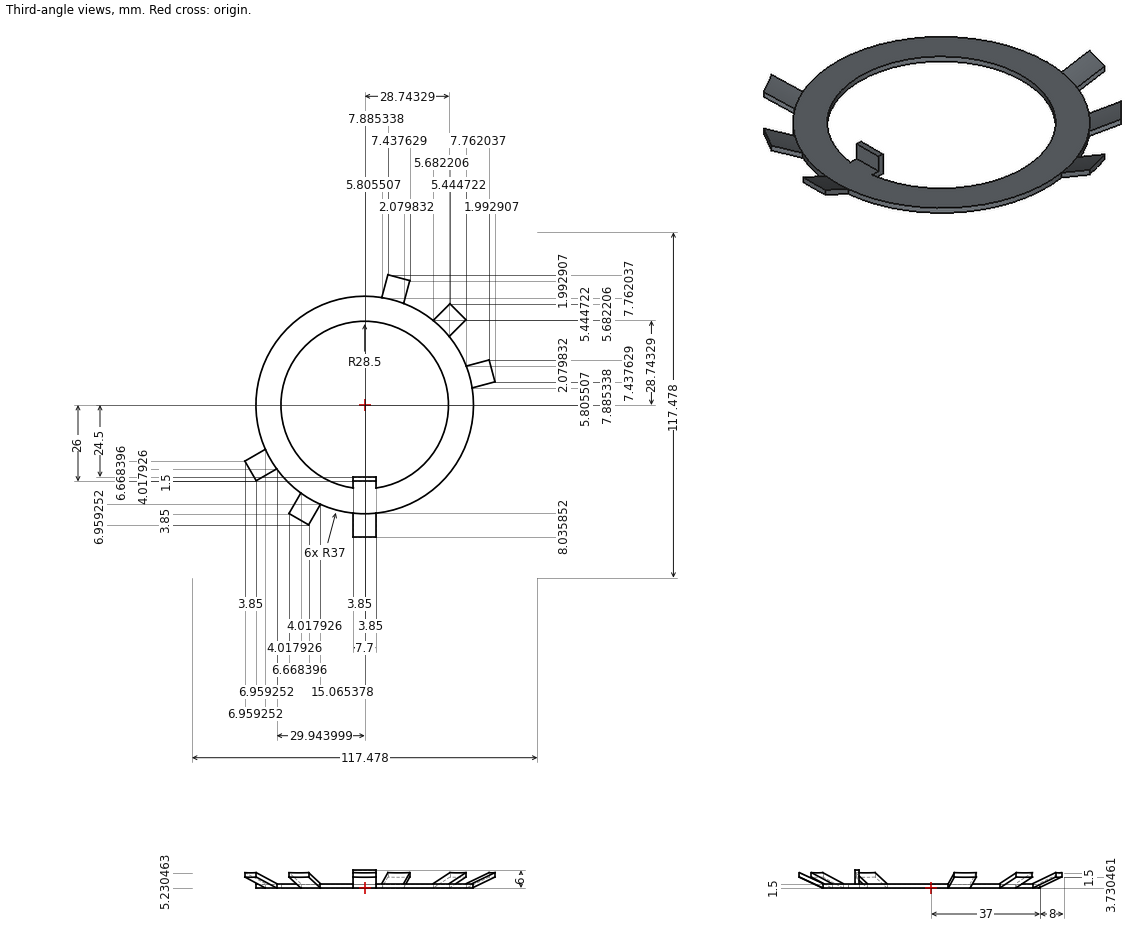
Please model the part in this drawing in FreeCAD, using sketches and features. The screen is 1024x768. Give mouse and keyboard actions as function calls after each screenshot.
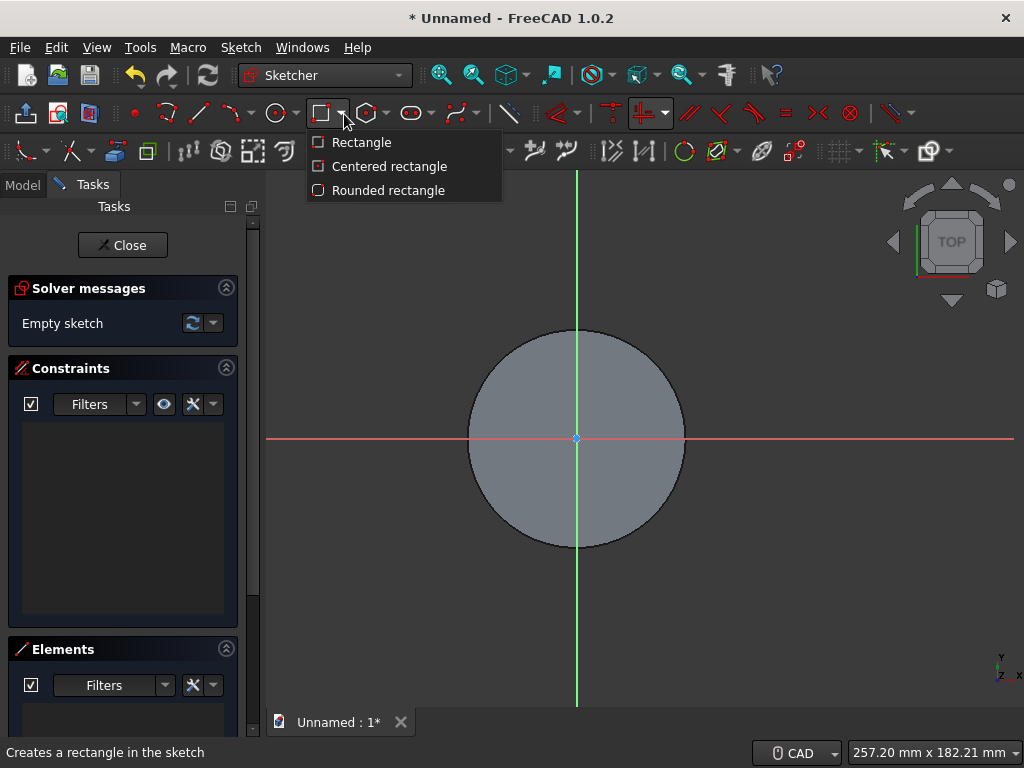
click(404, 166)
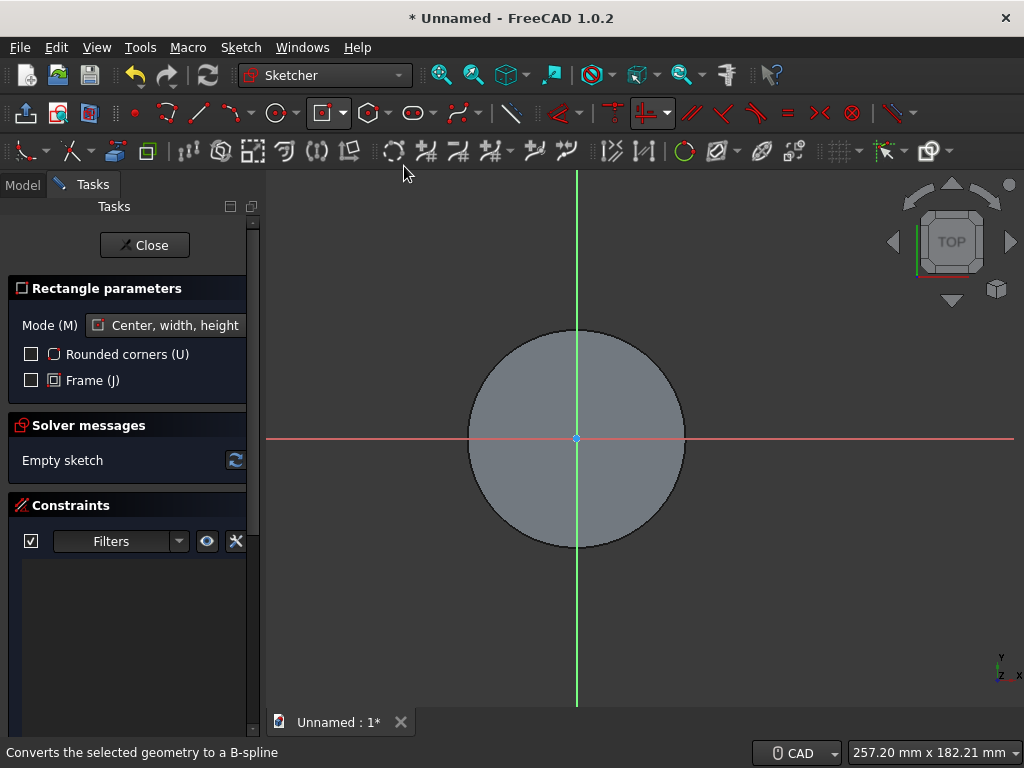
click(577, 439)
click(750, 266)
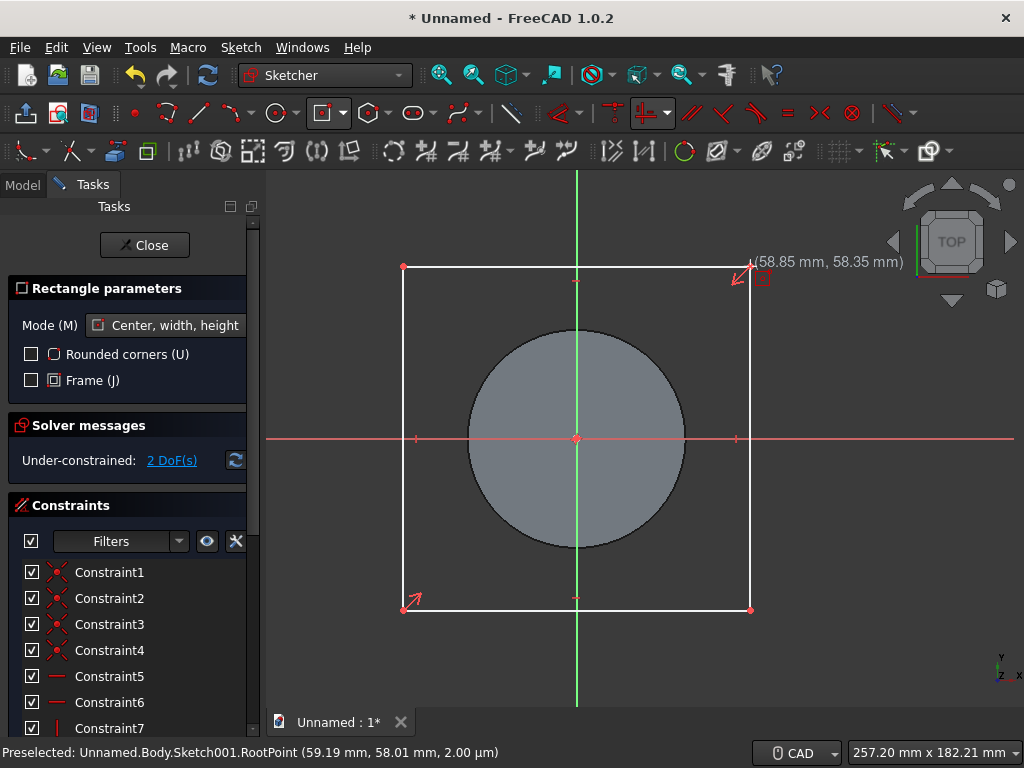
click(168, 114)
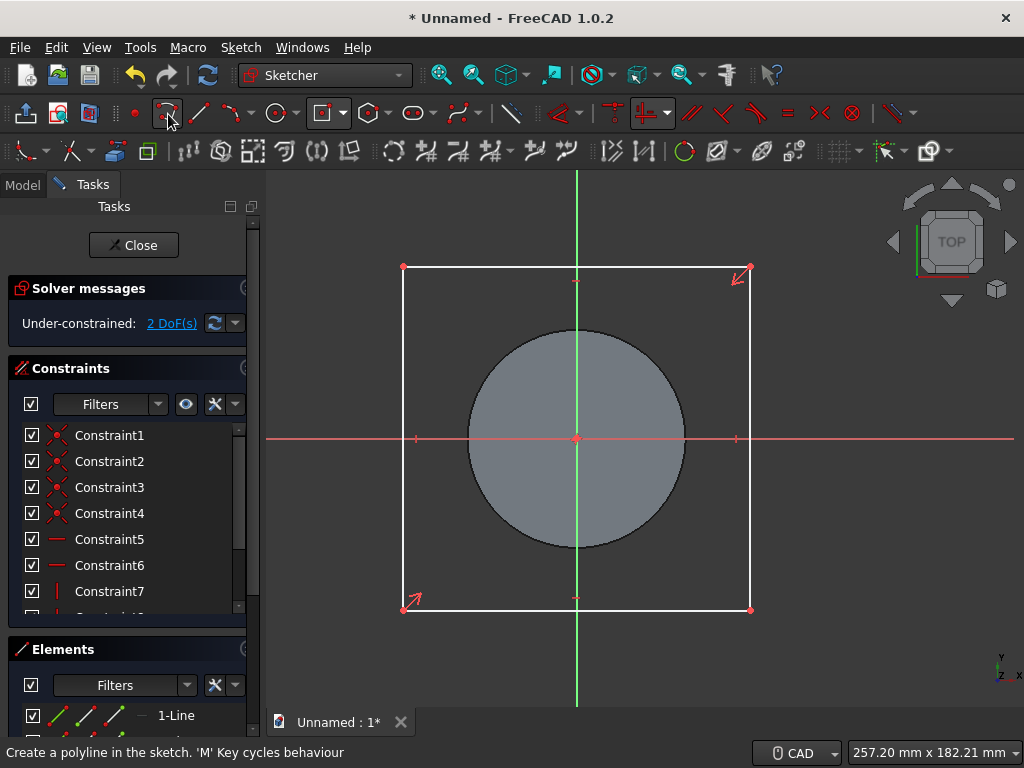
scroll(565, 522, up, 2)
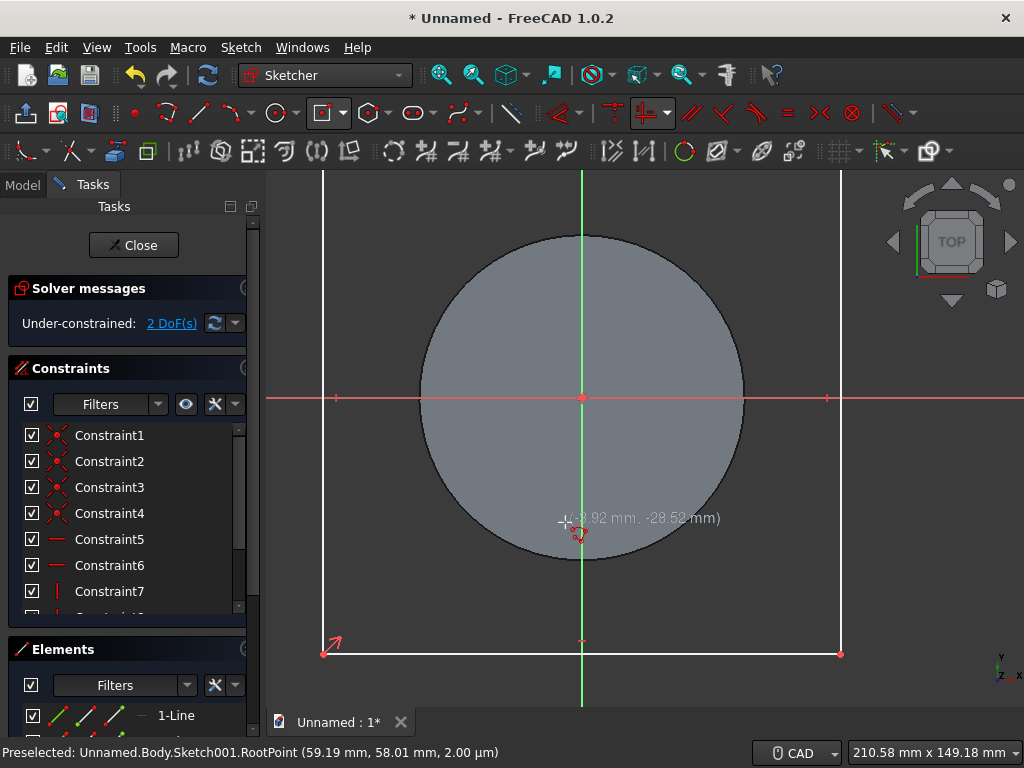
click(565, 522)
click(565, 506)
click(599, 506)
click(599, 522)
right_click(599, 522)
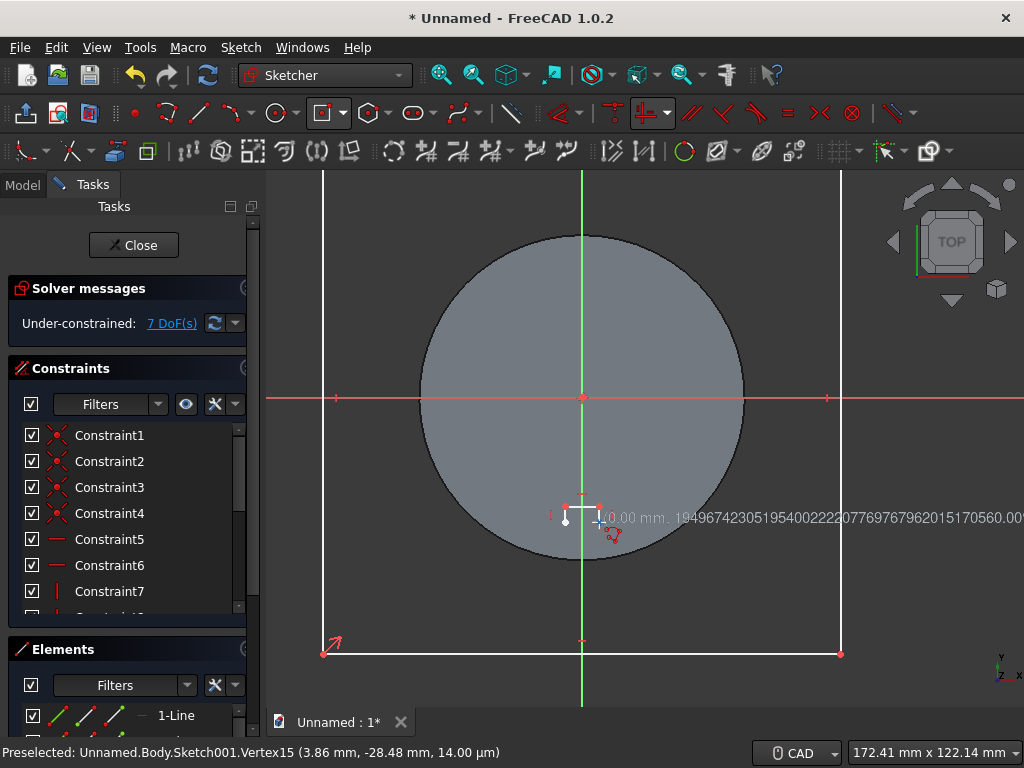
click(232, 114)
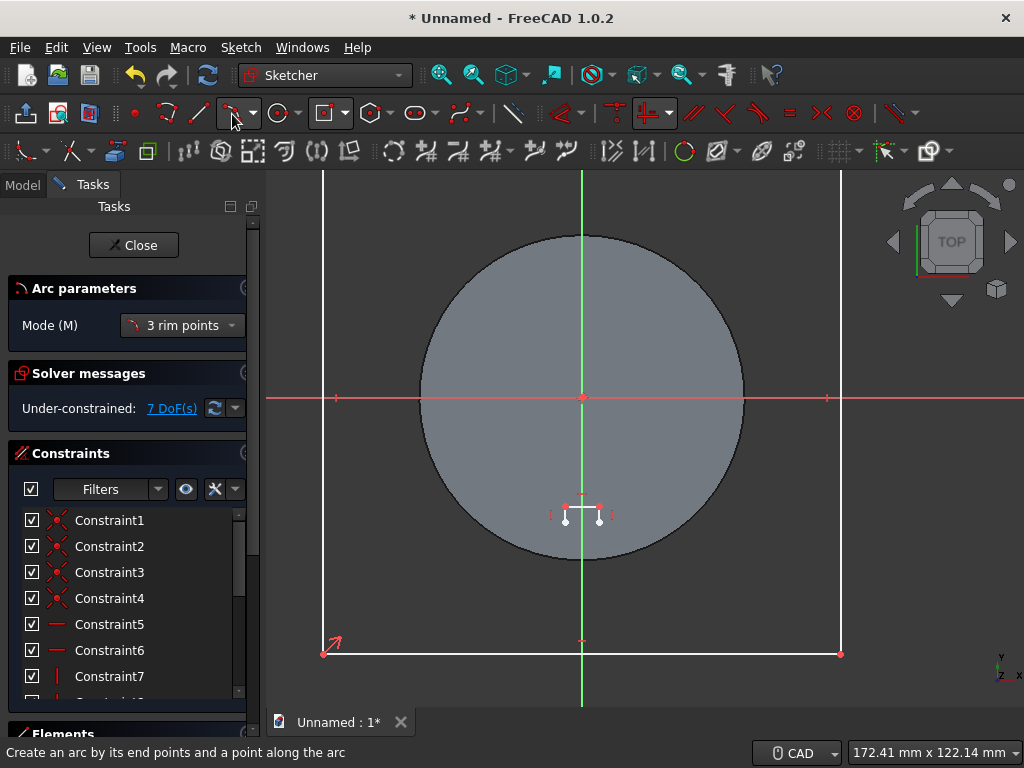
scroll(599, 522, up, 4)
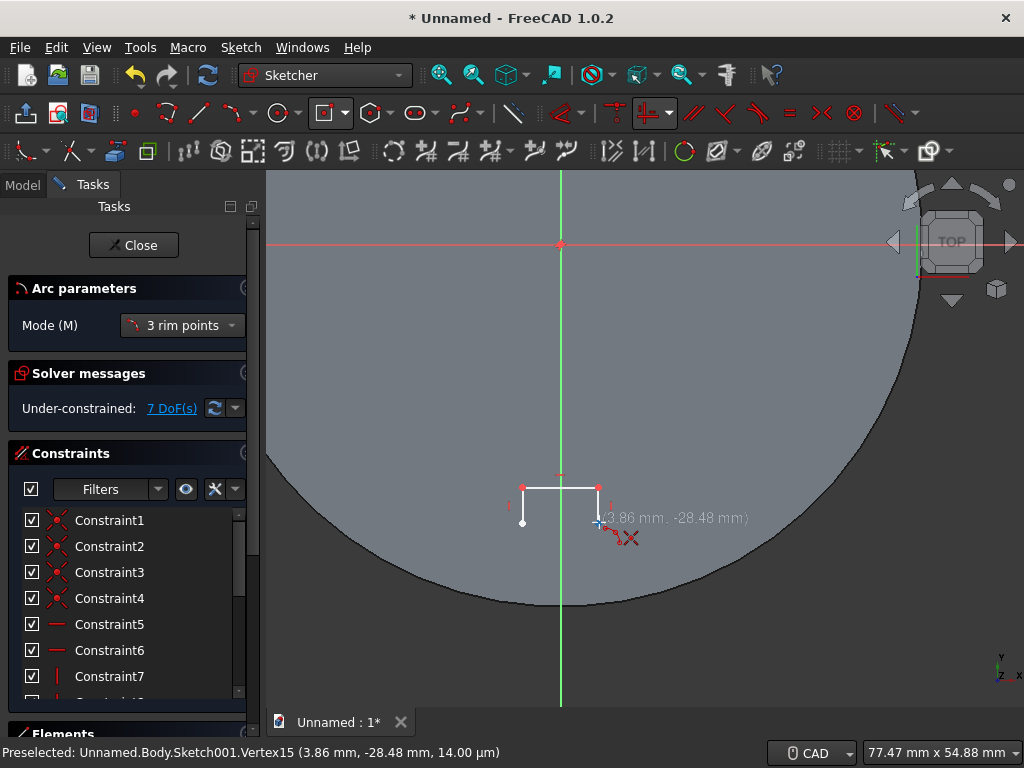
click(598, 523)
click(523, 523)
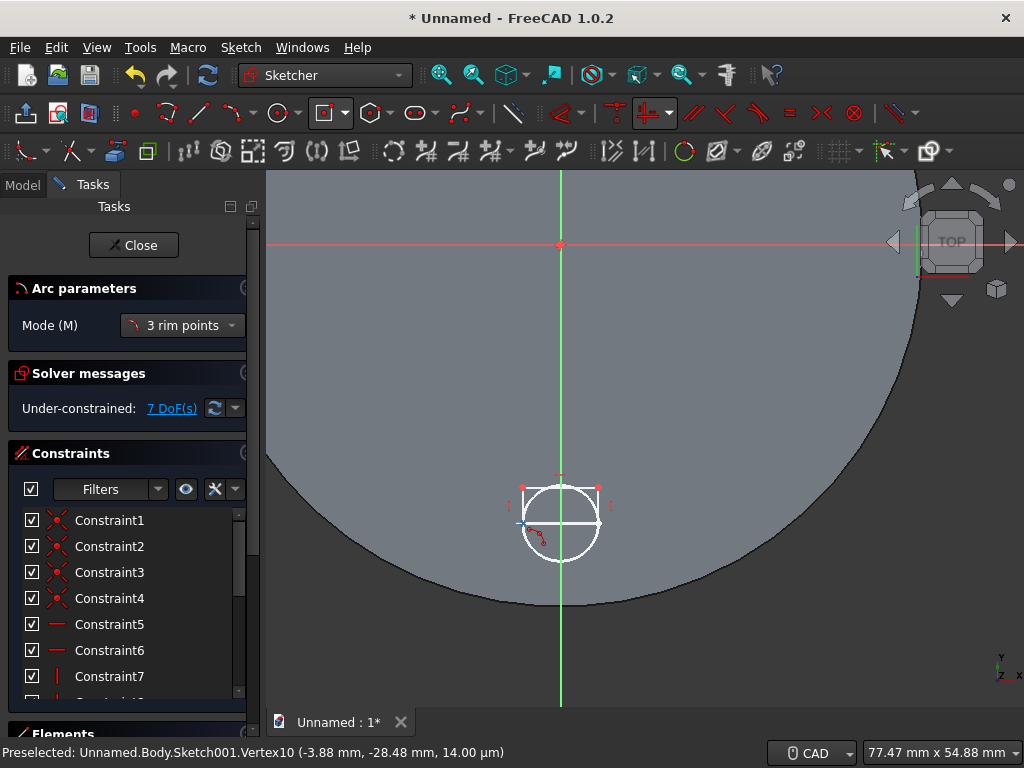
scroll(583, 522, down, 6)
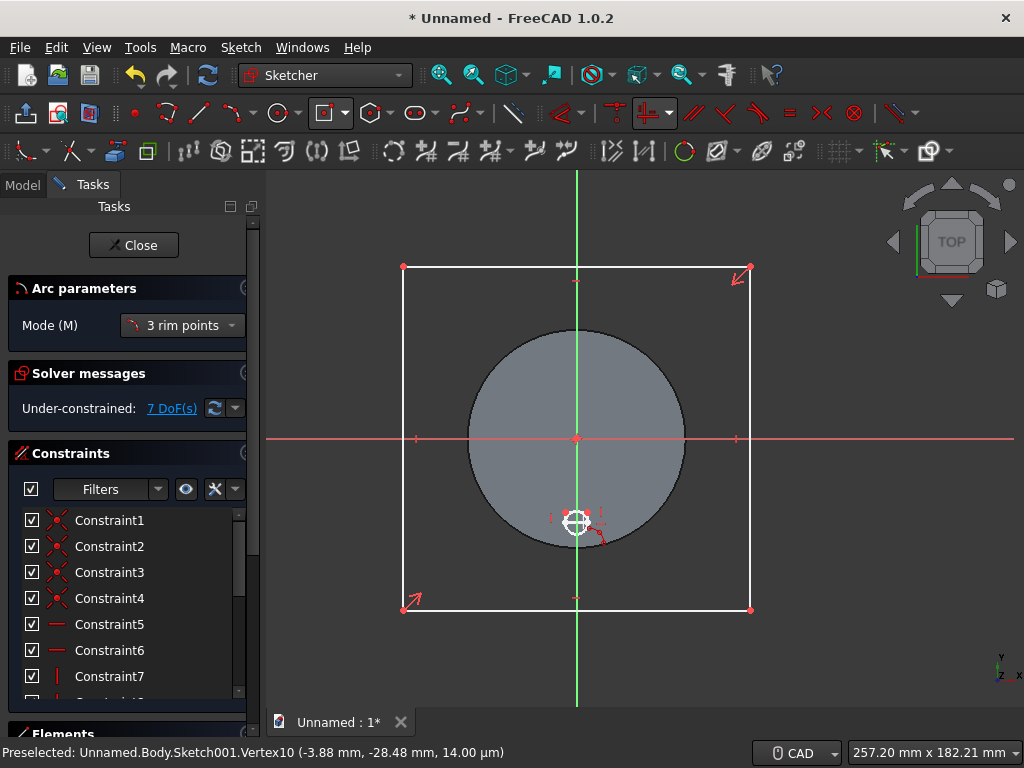
click(624, 370)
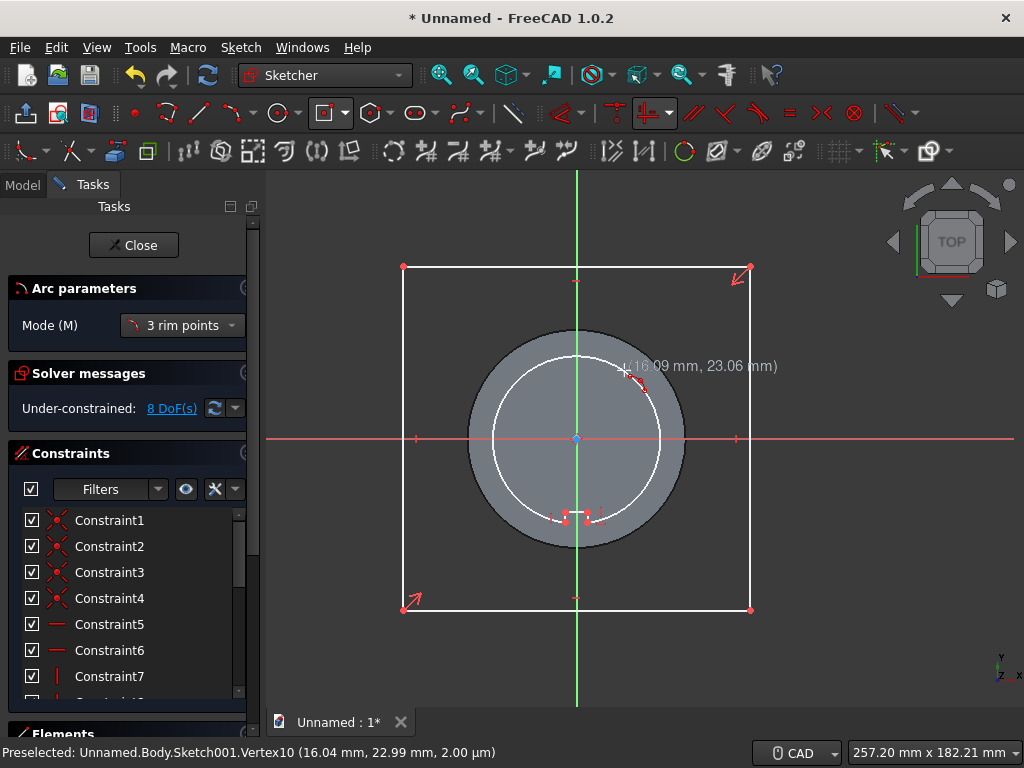
click(168, 114)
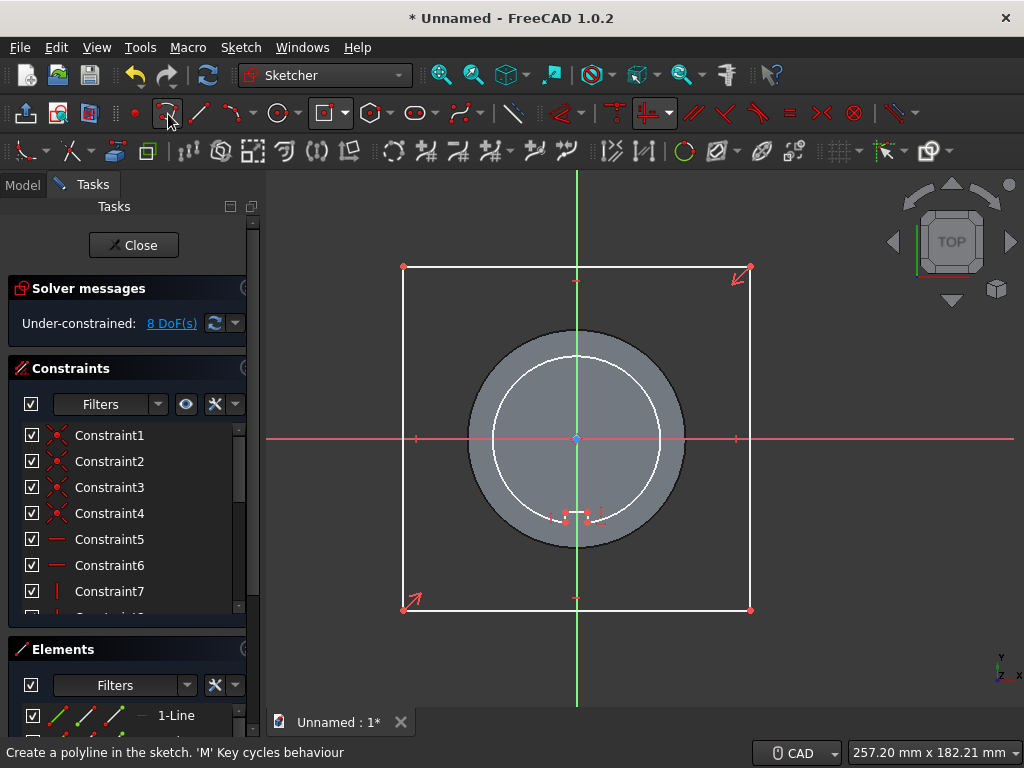
click(532, 539)
click(520, 559)
click(501, 548)
click(513, 527)
right_click(513, 527)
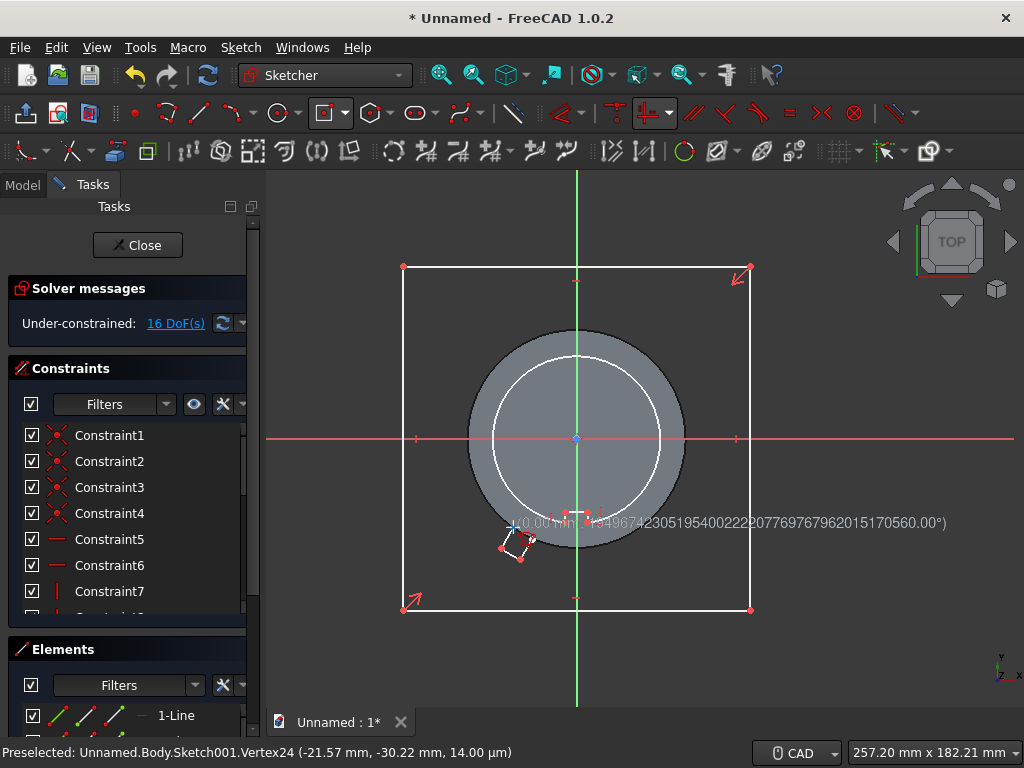
click(488, 503)
click(468, 515)
click(456, 495)
click(477, 483)
right_click(477, 483)